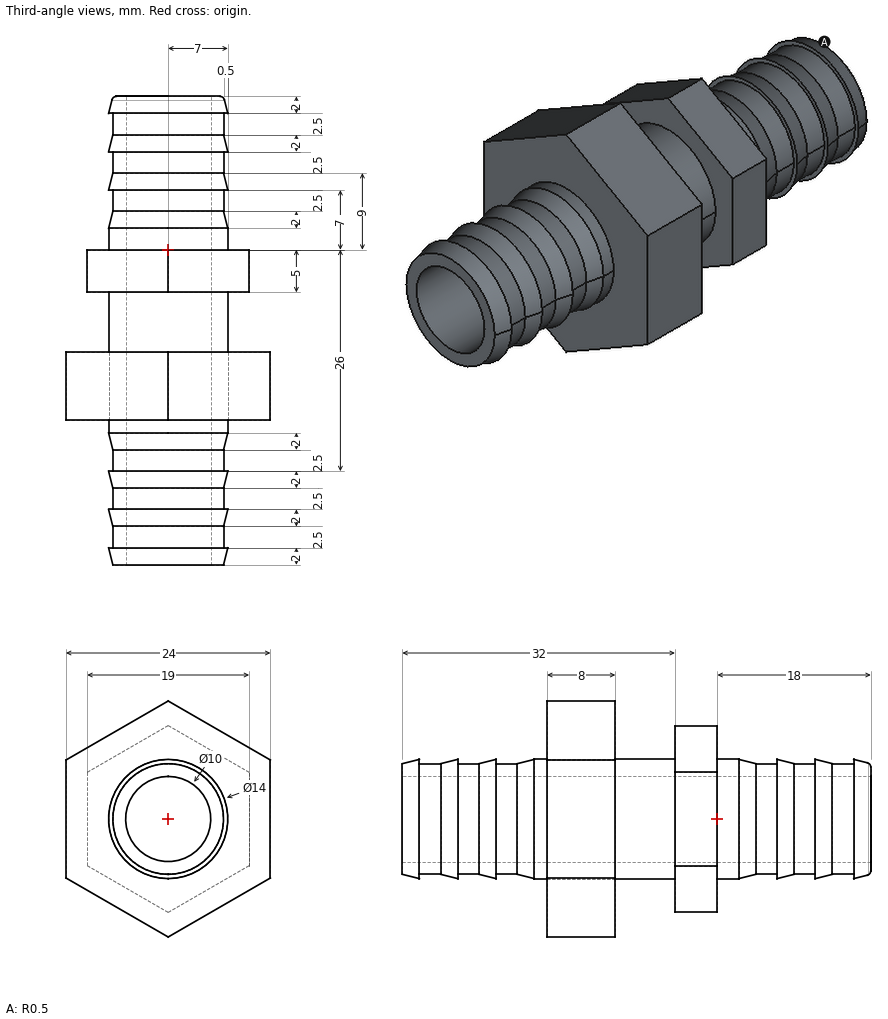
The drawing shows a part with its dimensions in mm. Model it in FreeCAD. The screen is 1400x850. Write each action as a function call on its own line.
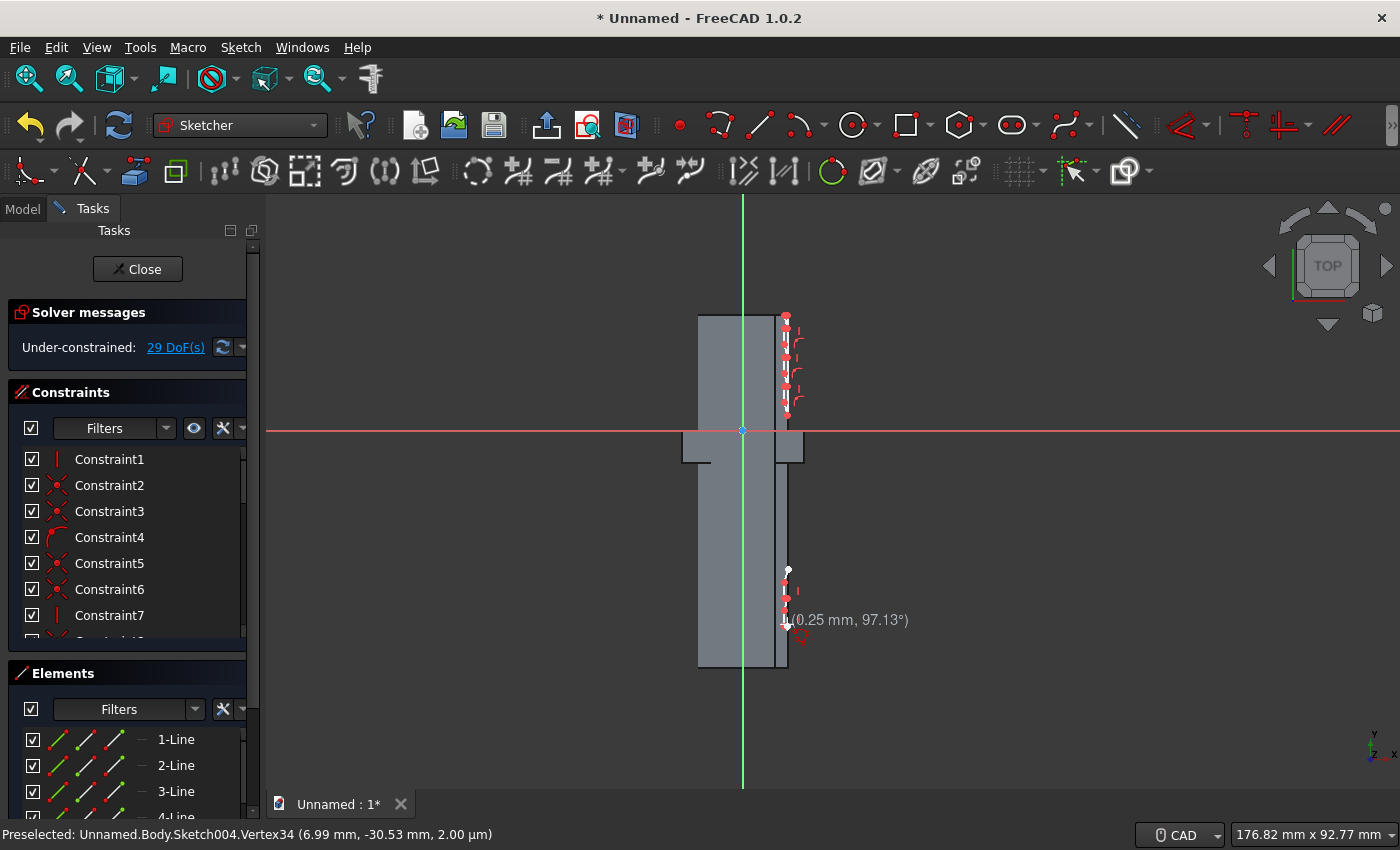
scroll(784, 639, up, 2)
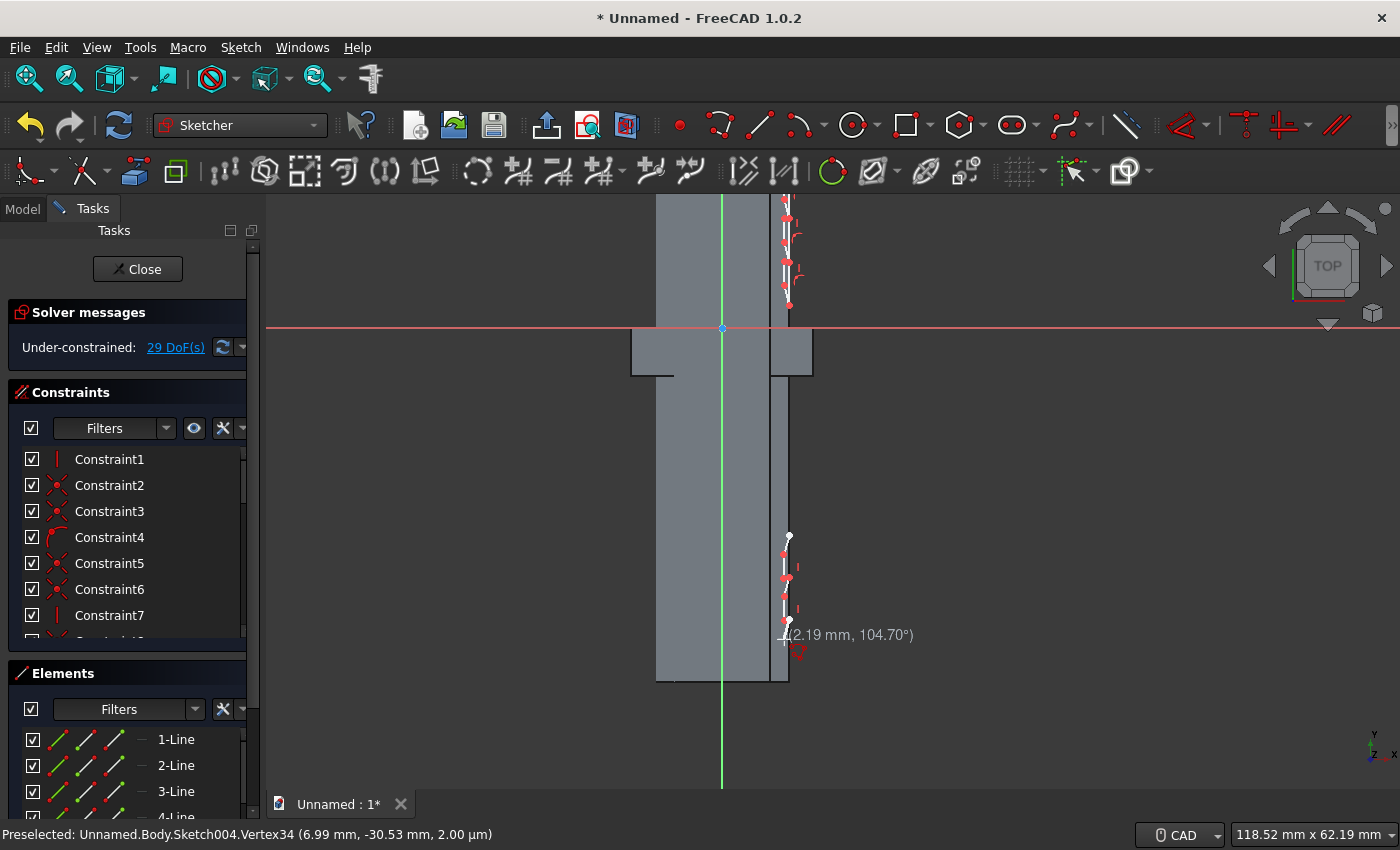
click(784, 639)
click(784, 663)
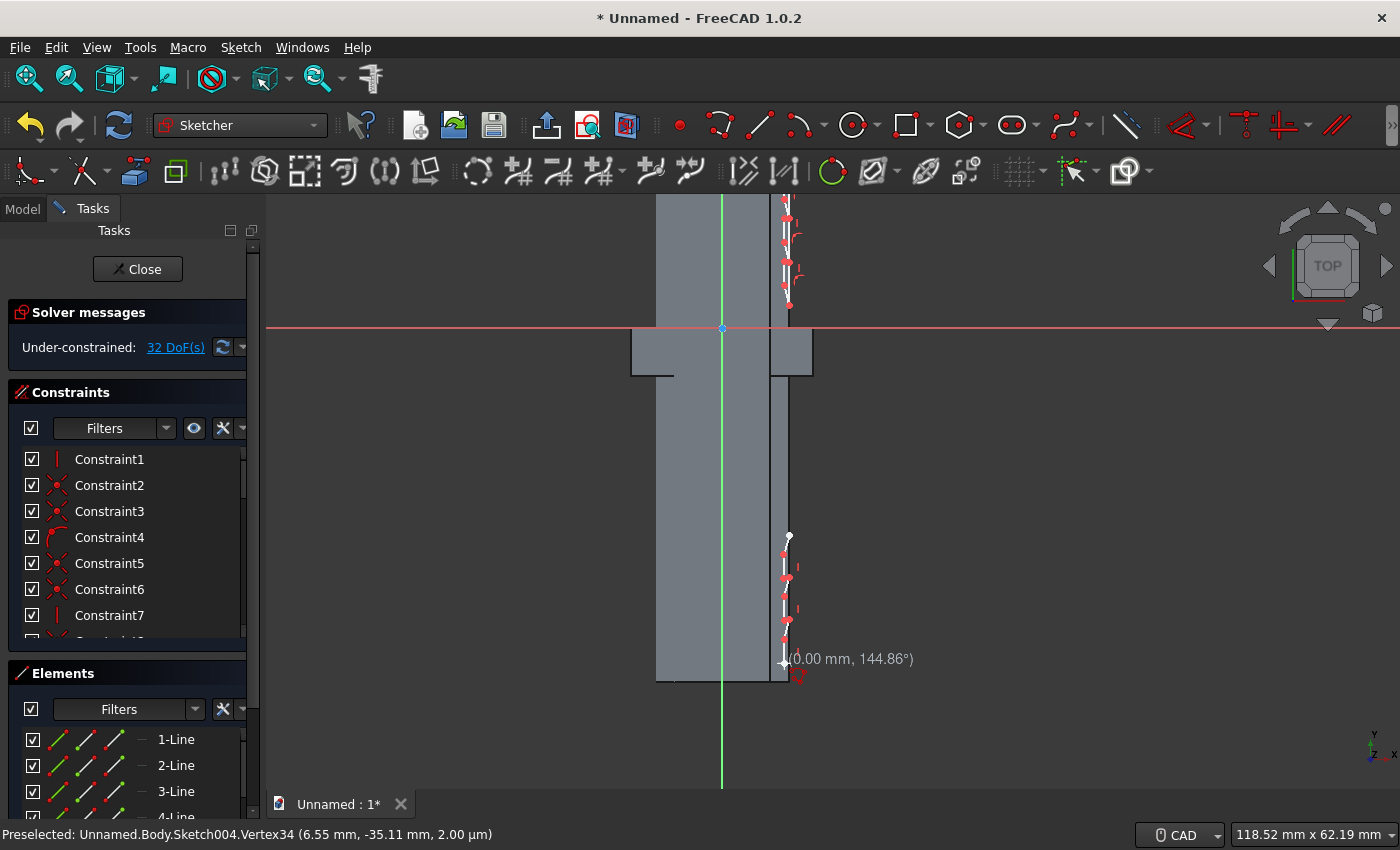
scroll(789, 663, up, 6)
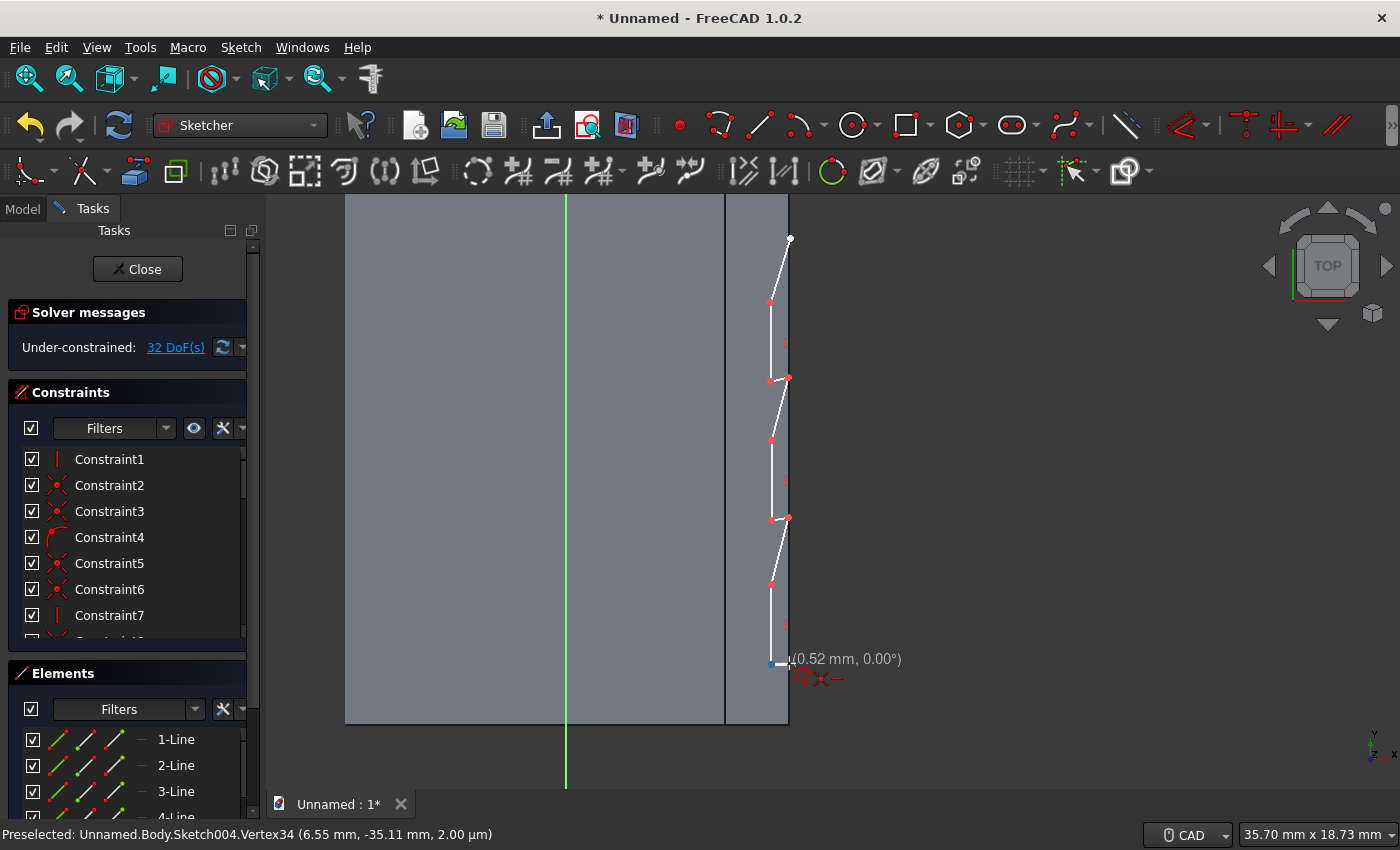
click(789, 661)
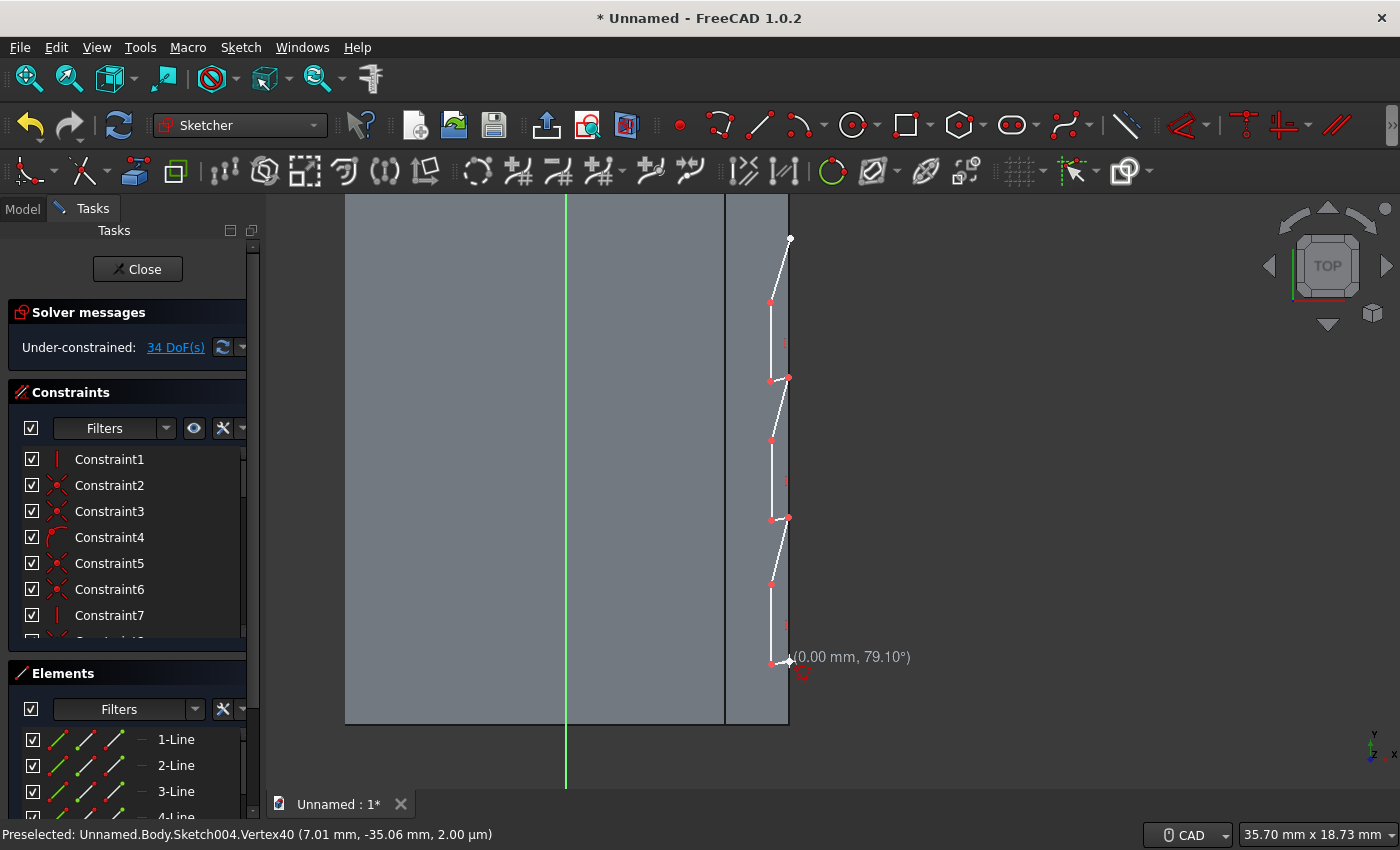
scroll(786, 654, down, 8)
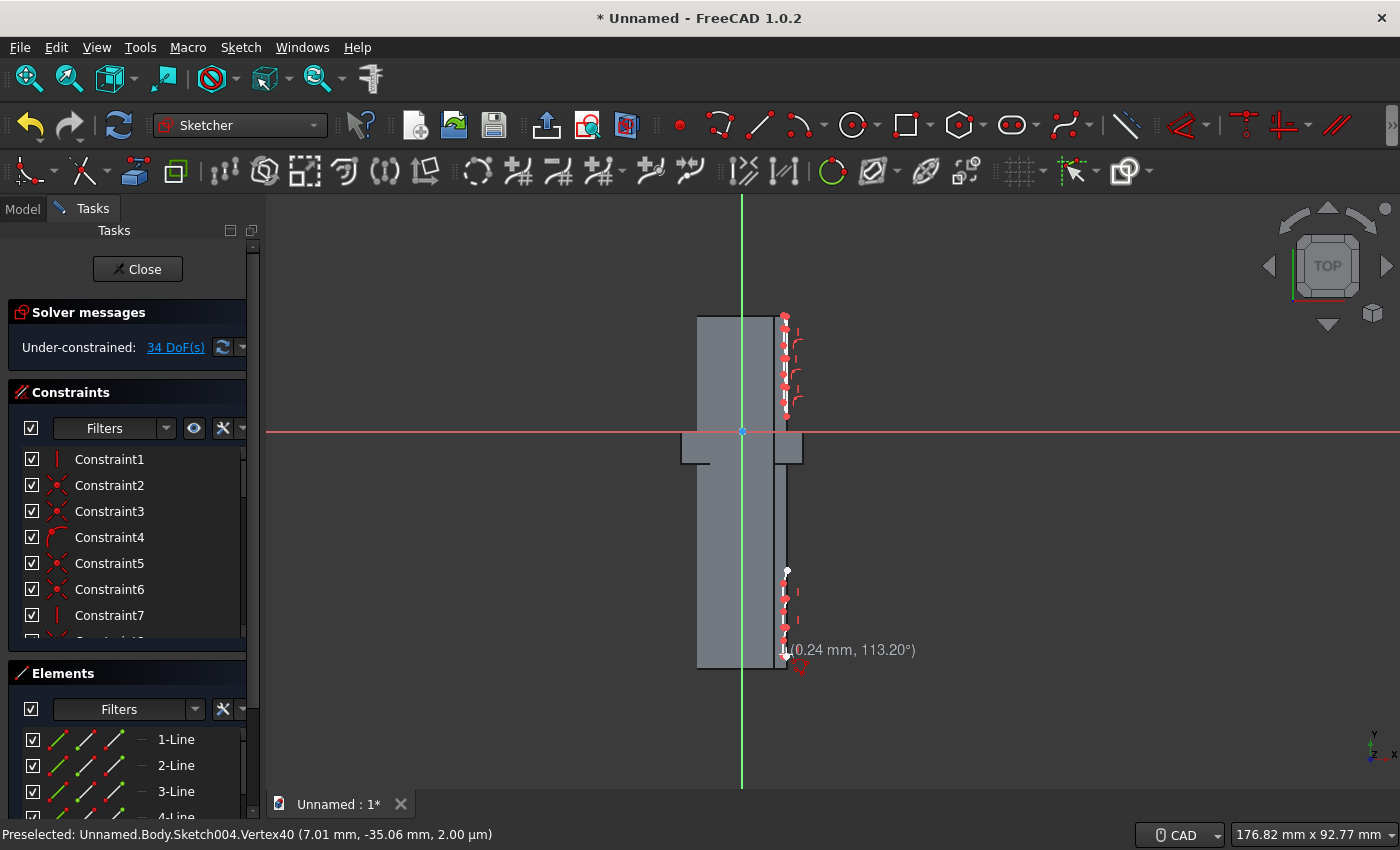
scroll(784, 669, up, 2)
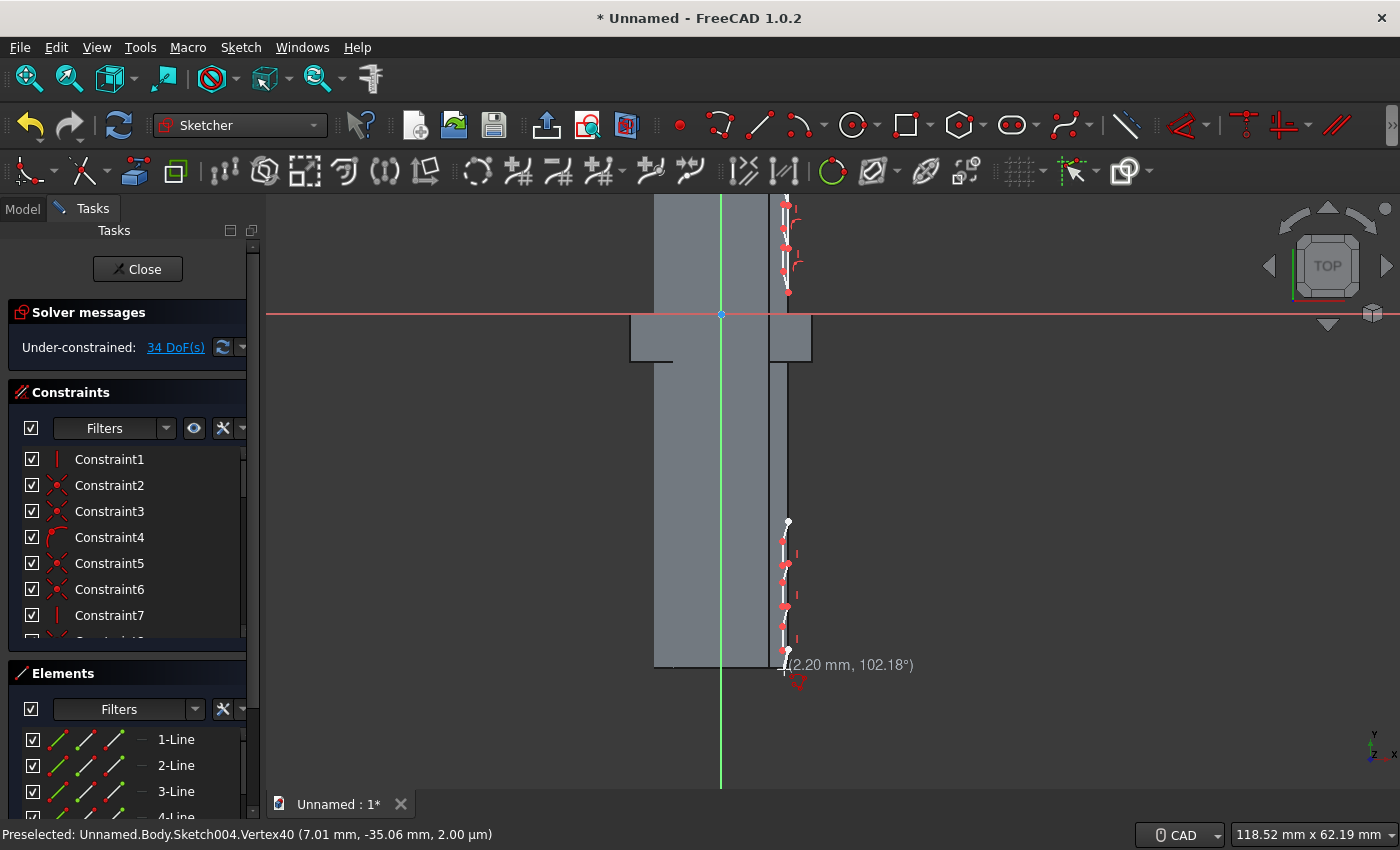
click(783, 668)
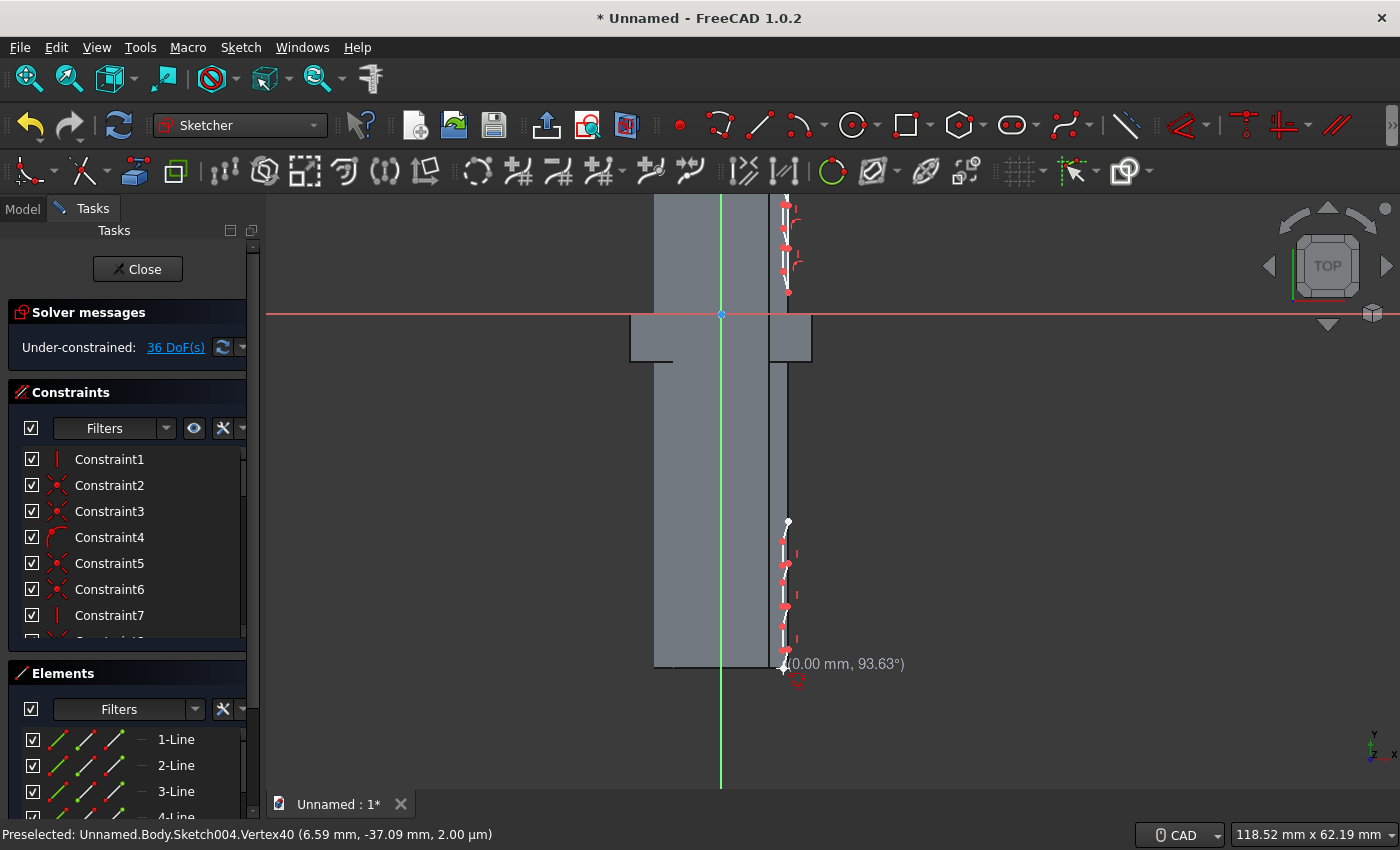
scroll(788, 668, up, 7)